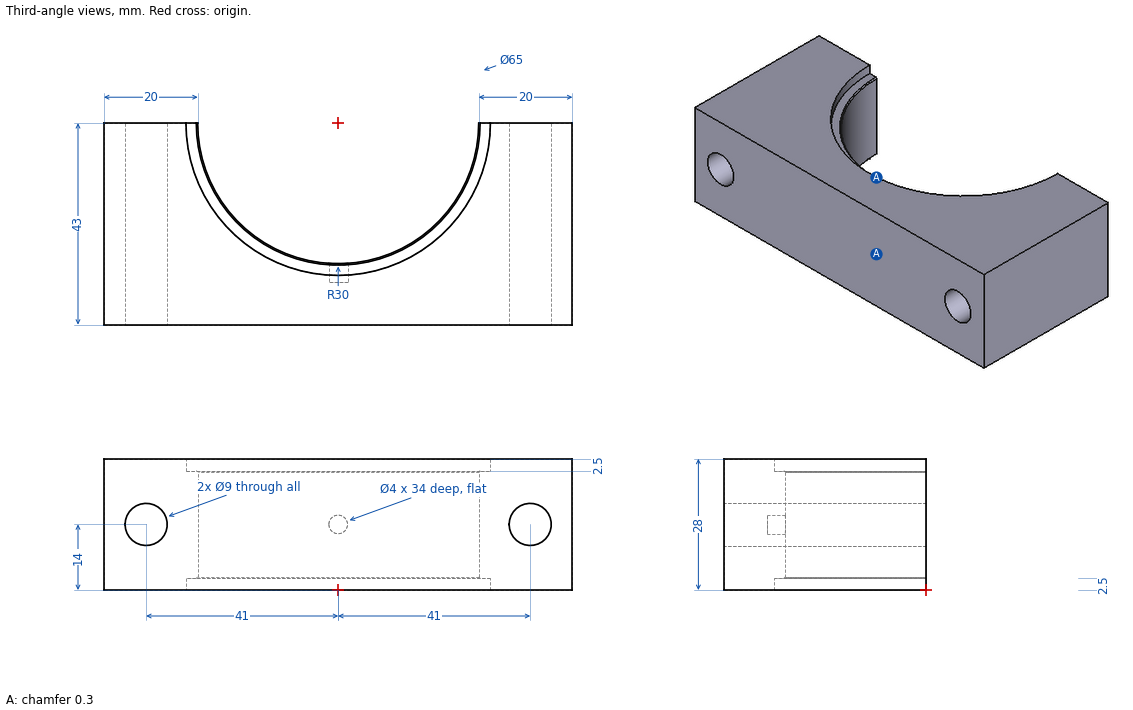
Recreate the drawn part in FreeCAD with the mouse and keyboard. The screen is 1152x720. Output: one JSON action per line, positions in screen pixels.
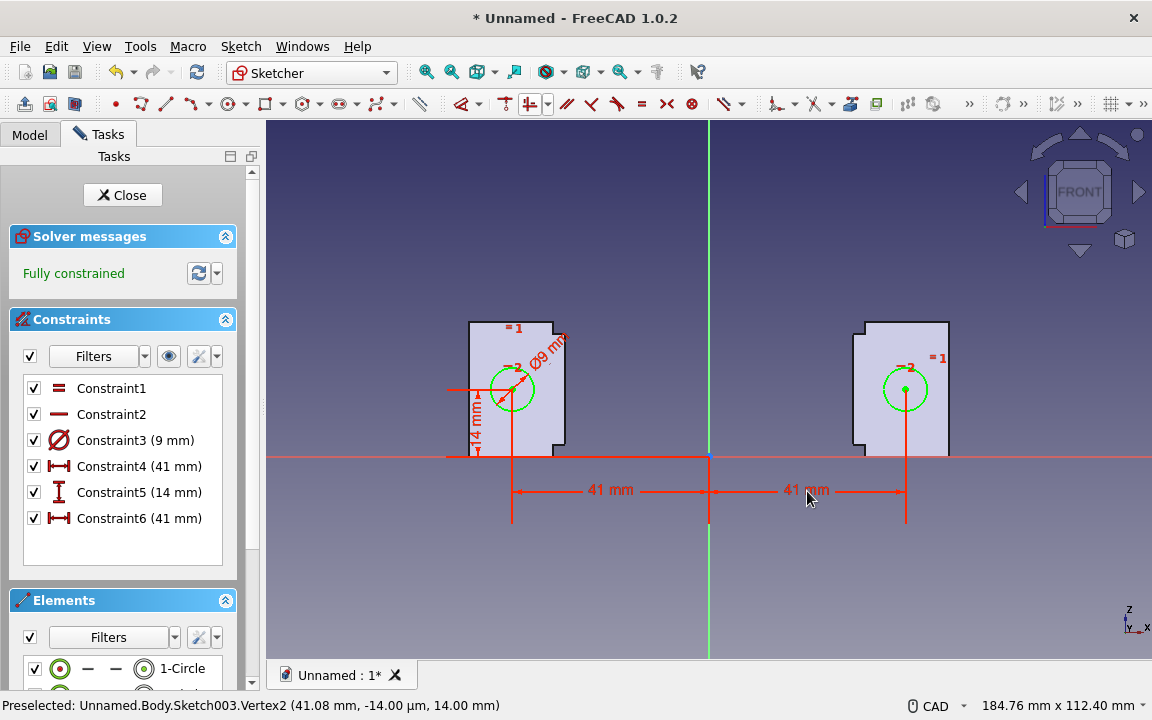
{"action": "left_click", "coordinate": [123, 195]}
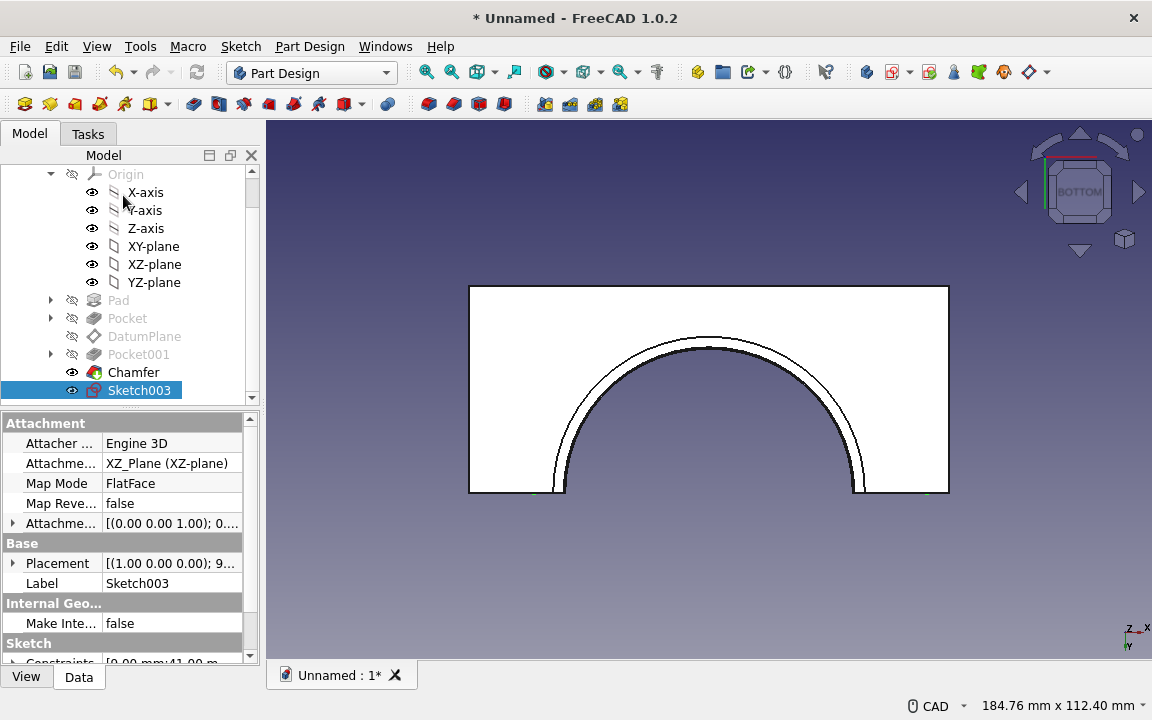
{"action": "left_click", "coordinate": [219, 104]}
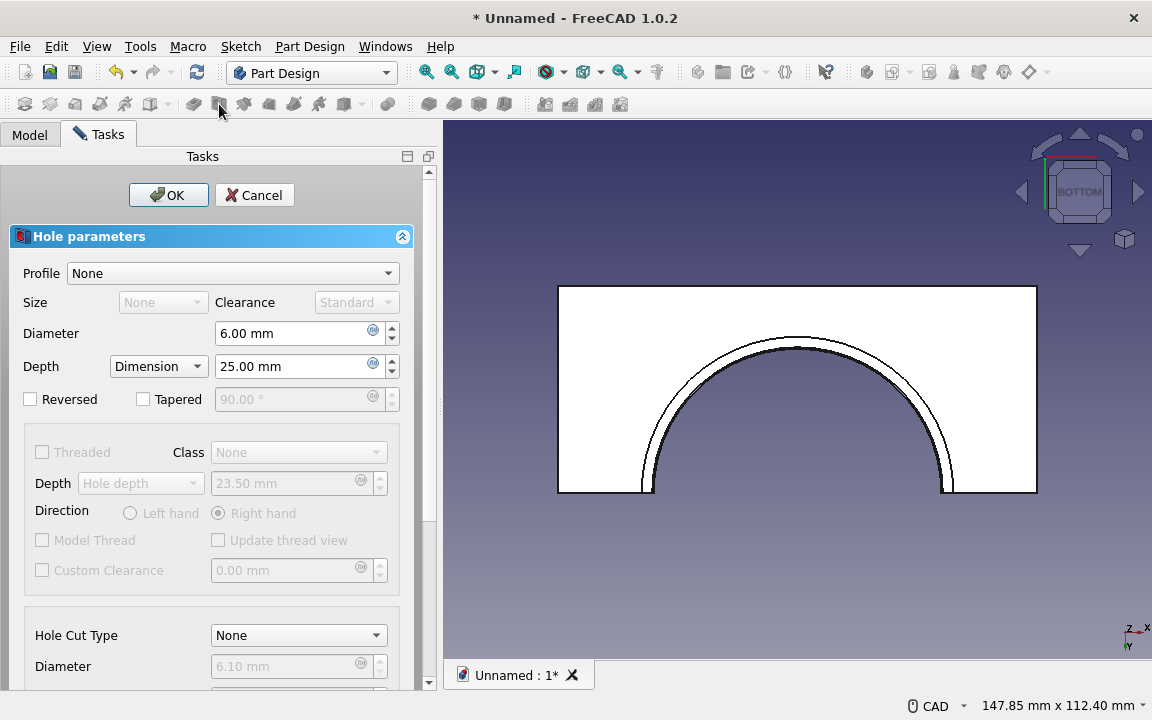
{"action": "triple_click", "coordinate": [300, 334]}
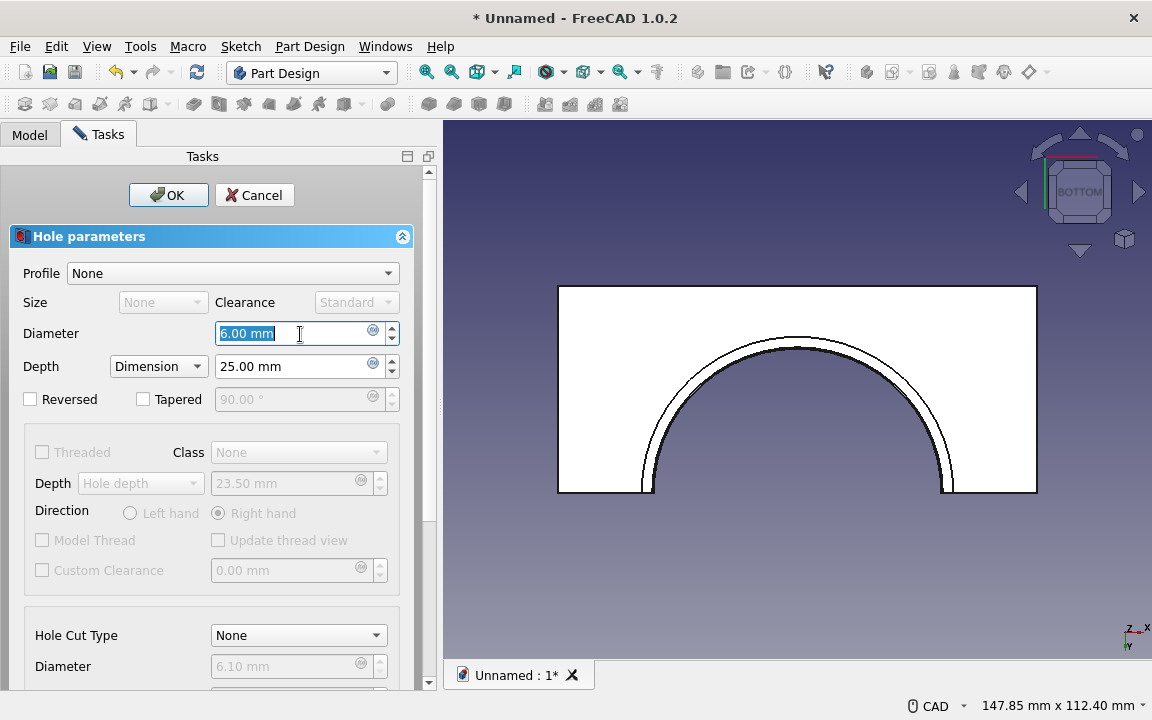
{"action": "type", "text": "9"}
{"action": "key", "text": "Tab"}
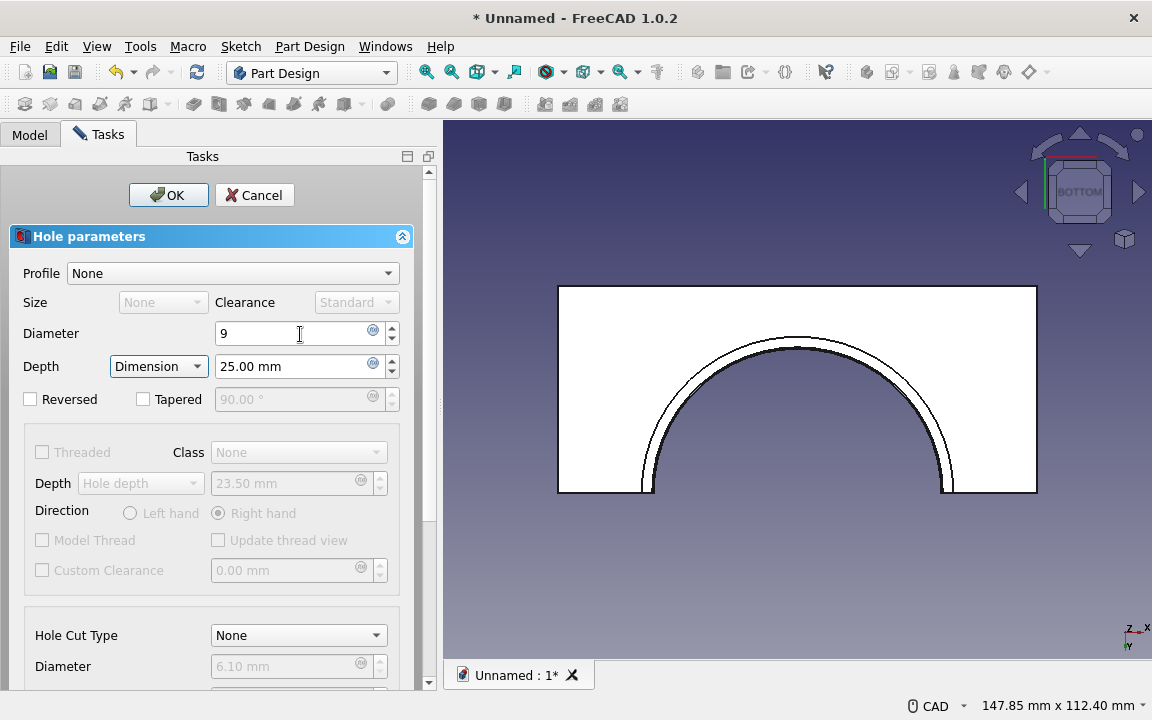
{"action": "left_click", "coordinate": [160, 366]}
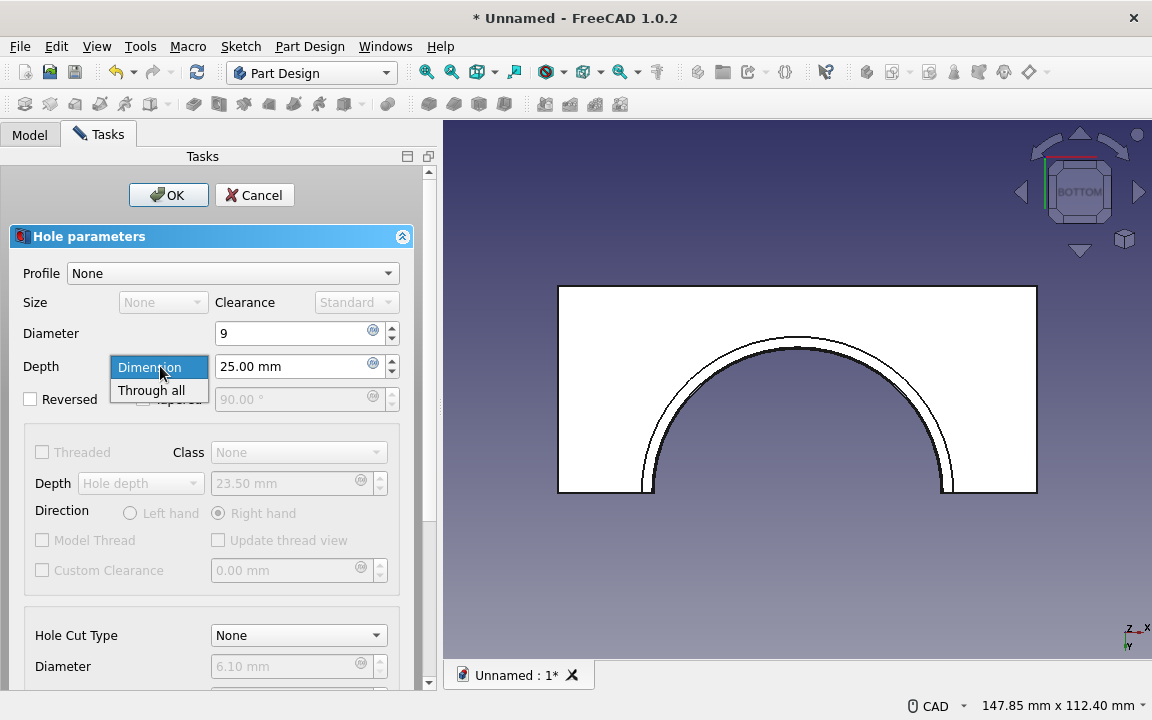
{"action": "left_click", "coordinate": [158, 390]}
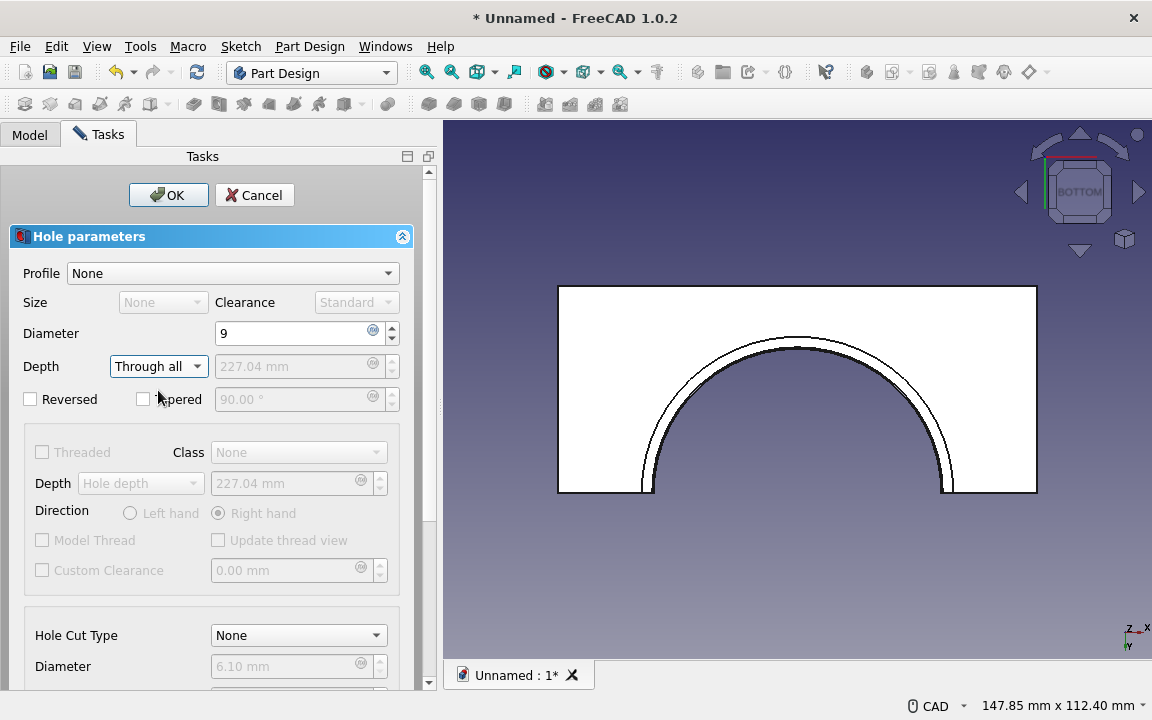
{"action": "left_click", "coordinate": [31, 399]}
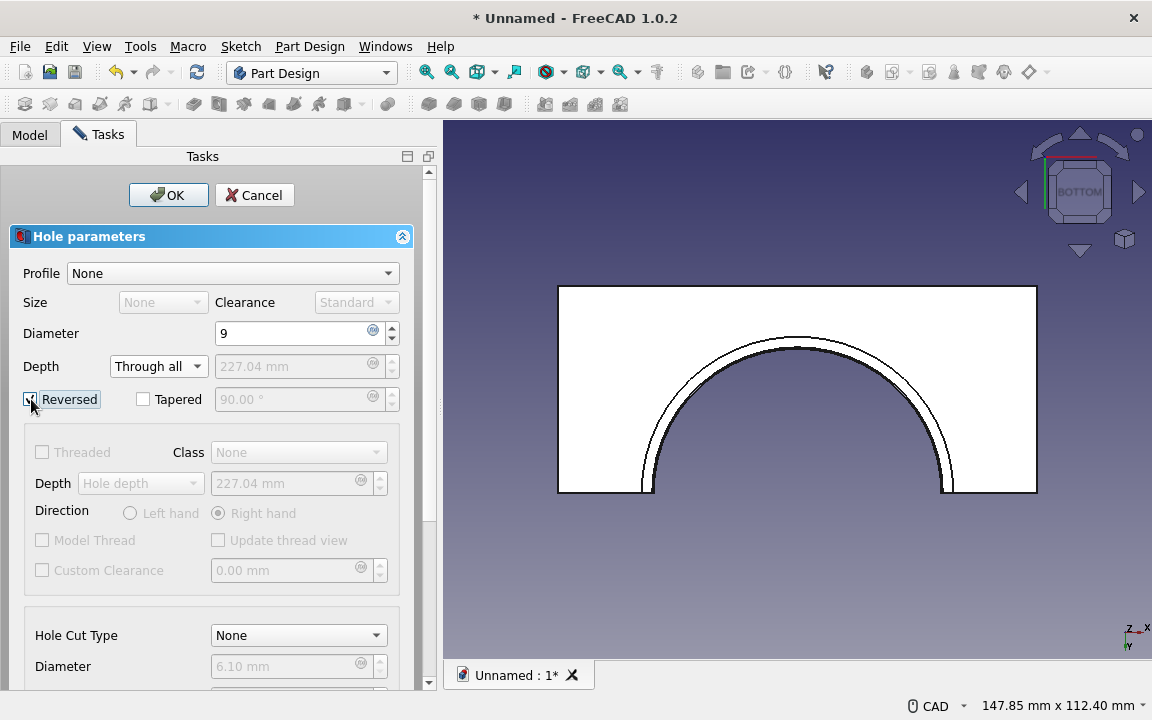
{"action": "left_click", "coordinate": [169, 195]}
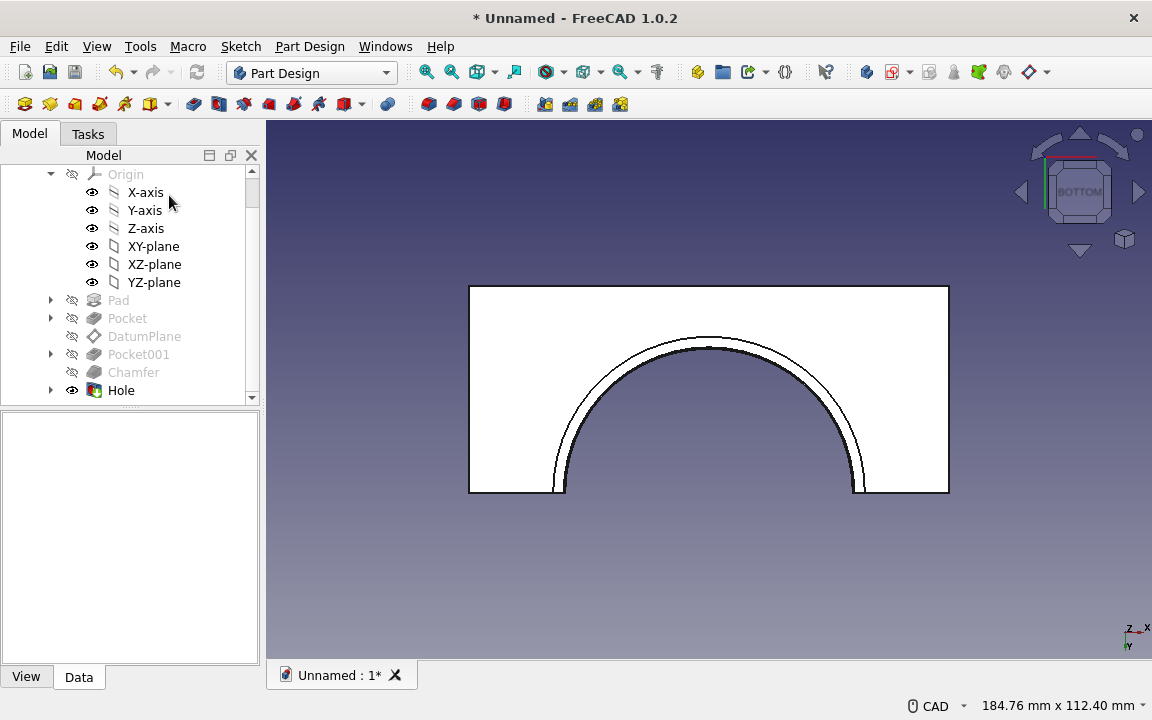
{"action": "key", "text": "4"}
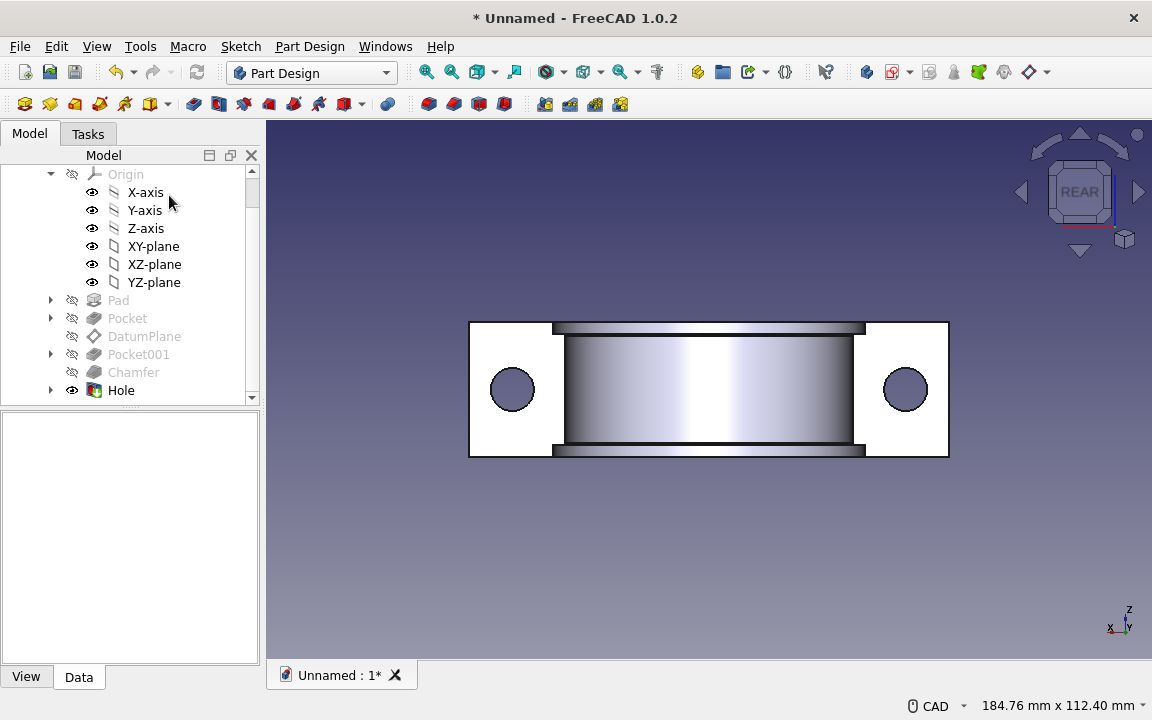
{"action": "left_click", "coordinate": [887, 350]}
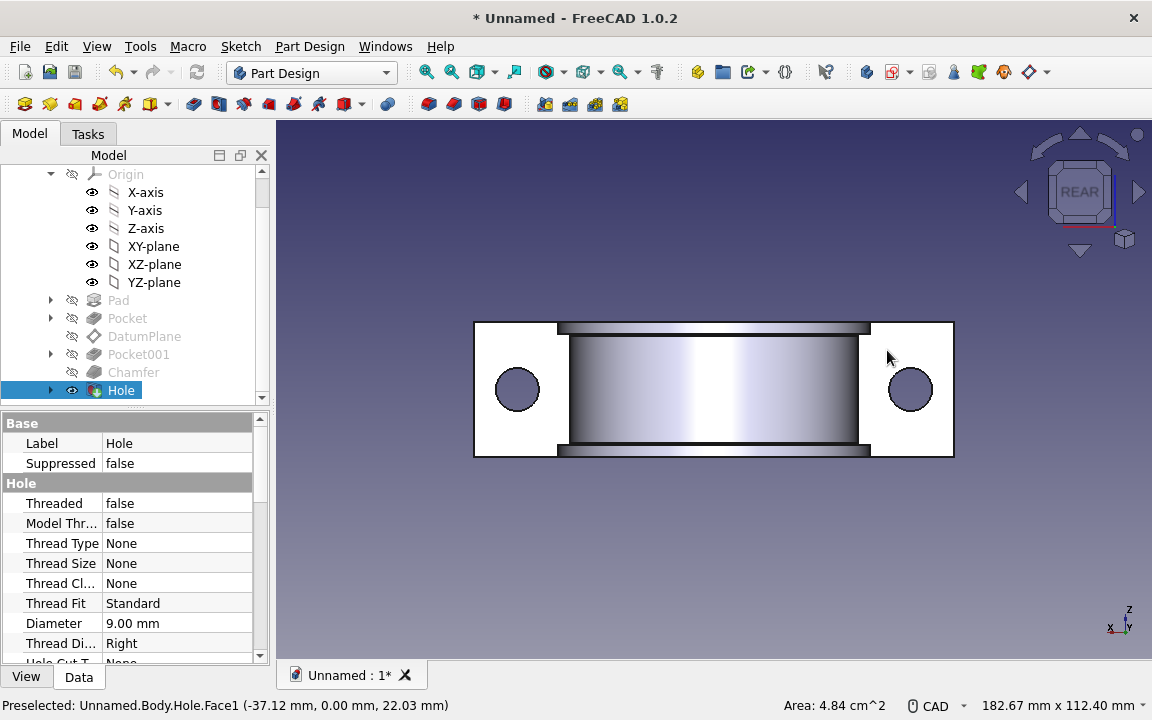
{"action": "left_click", "coordinate": [892, 72]}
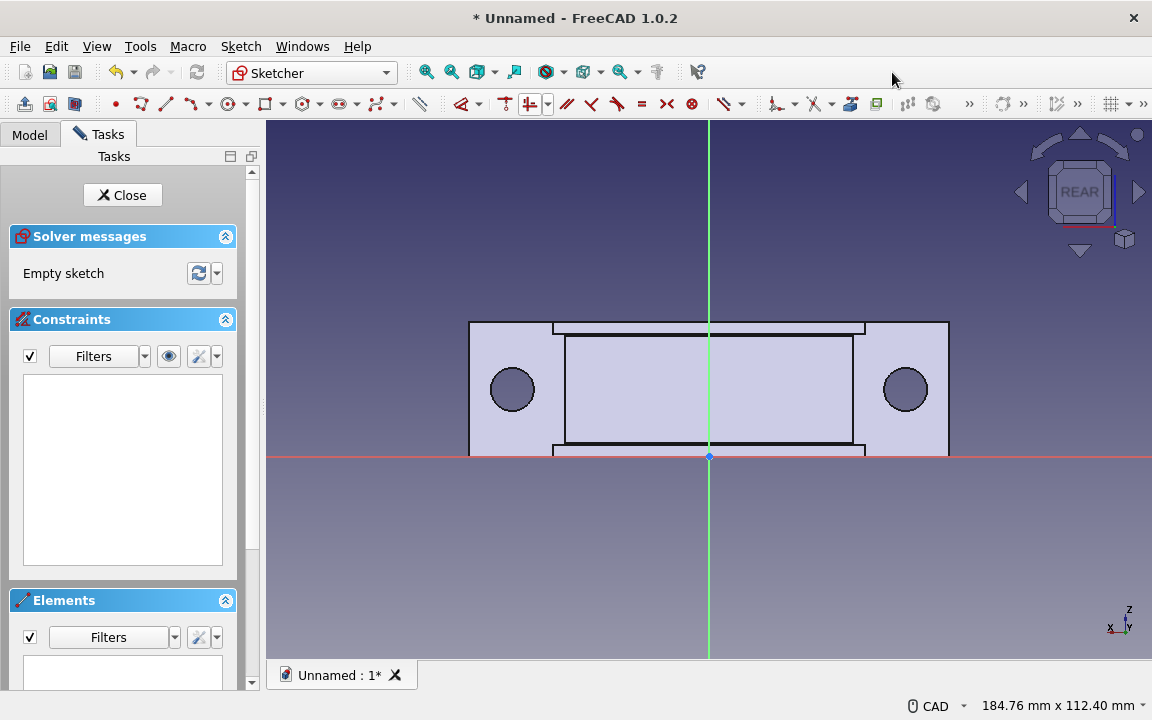
{"action": "scroll", "coordinate": [713, 389], "scroll_direction": "up", "scroll_amount": 14}